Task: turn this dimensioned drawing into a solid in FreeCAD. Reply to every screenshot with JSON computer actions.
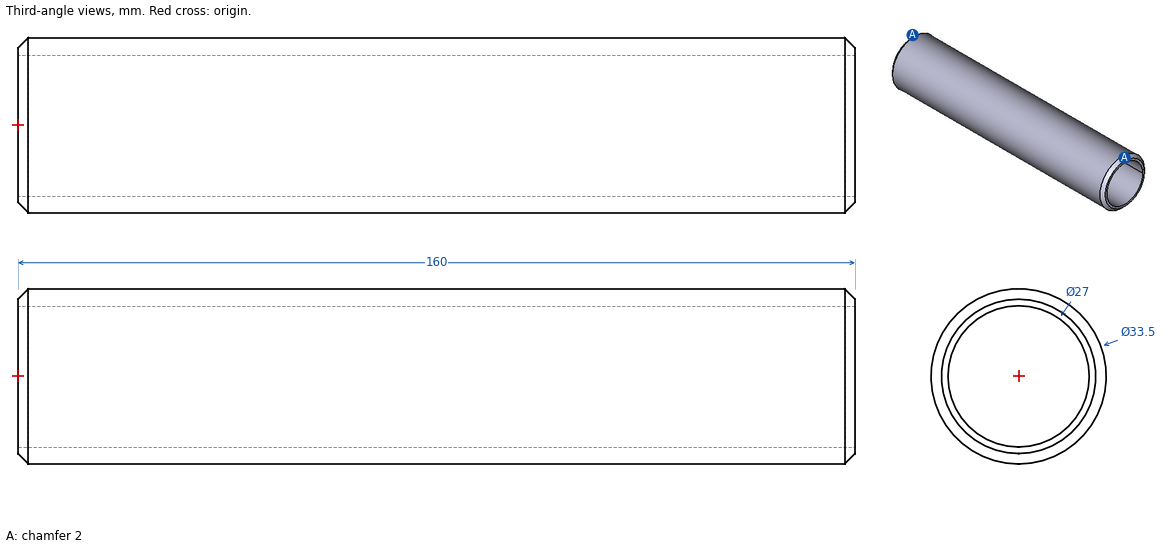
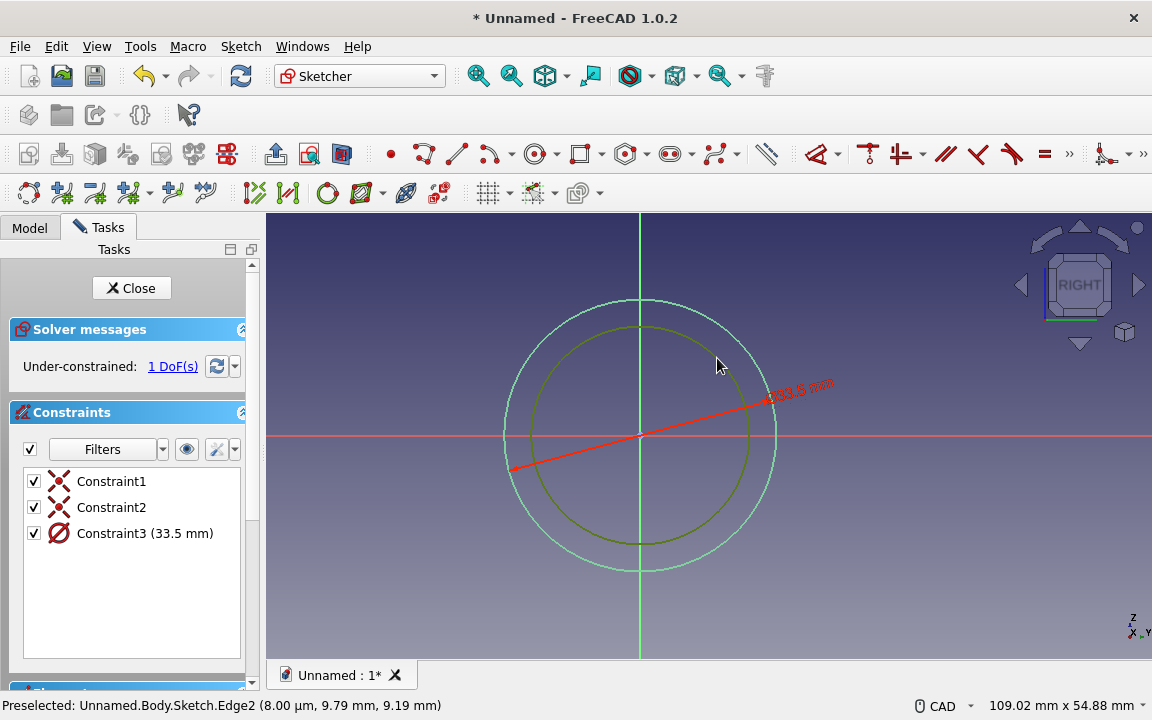
{"action": "key", "text": "k o"}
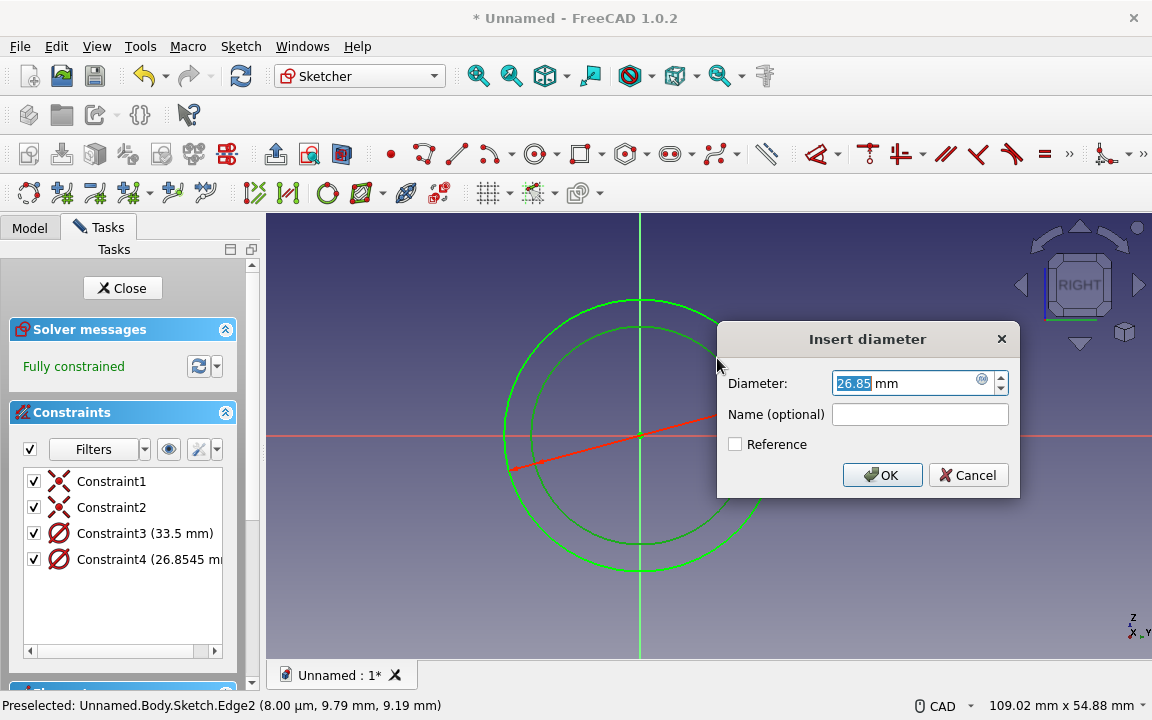
{"action": "type", "text": "27"}
{"action": "key", "text": "Return"}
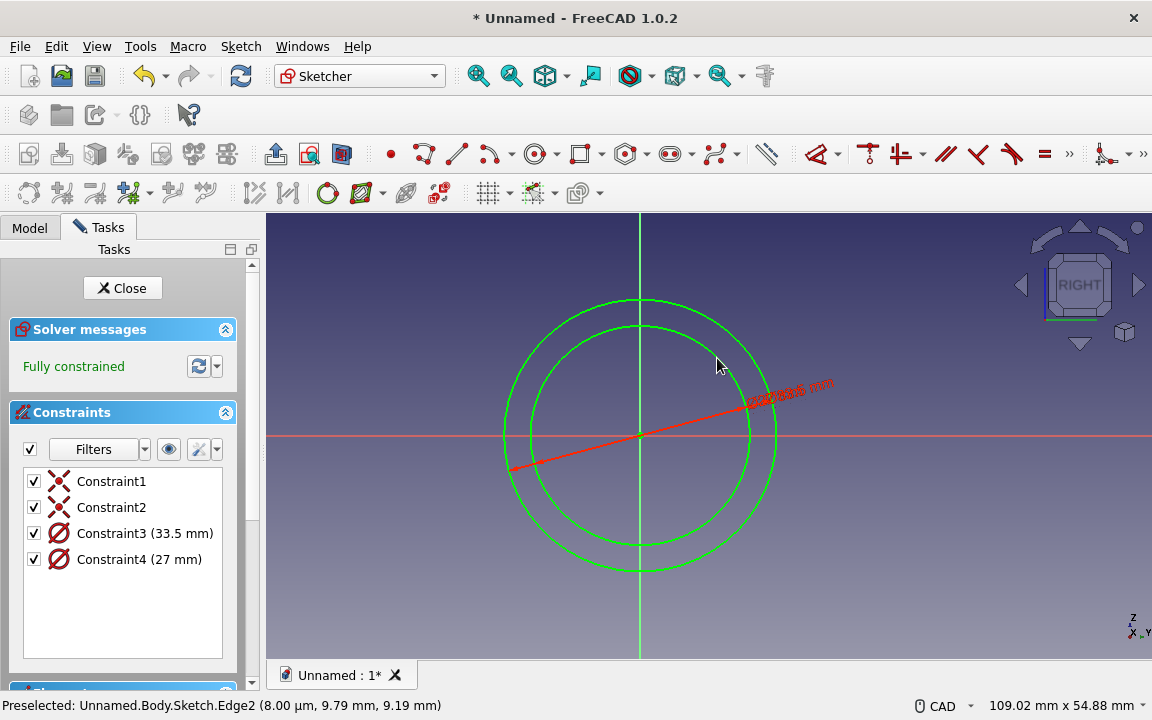
{"action": "left_click", "coordinate": [123, 288]}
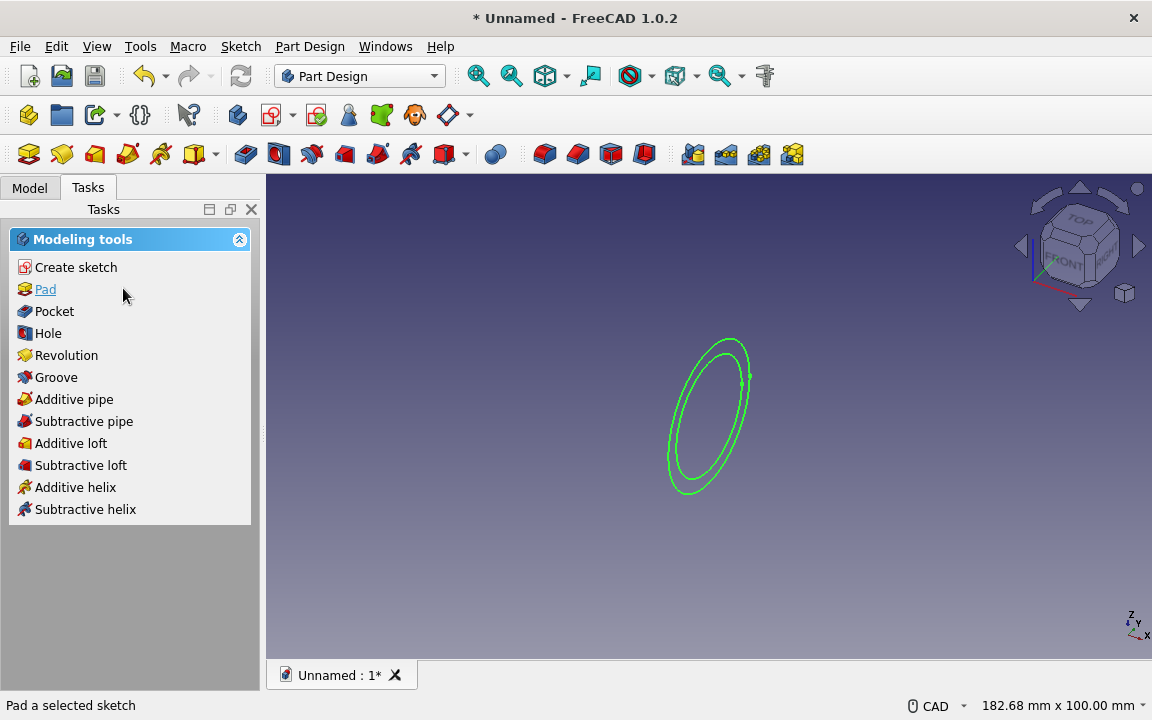
{"action": "left_click", "coordinate": [29, 154]}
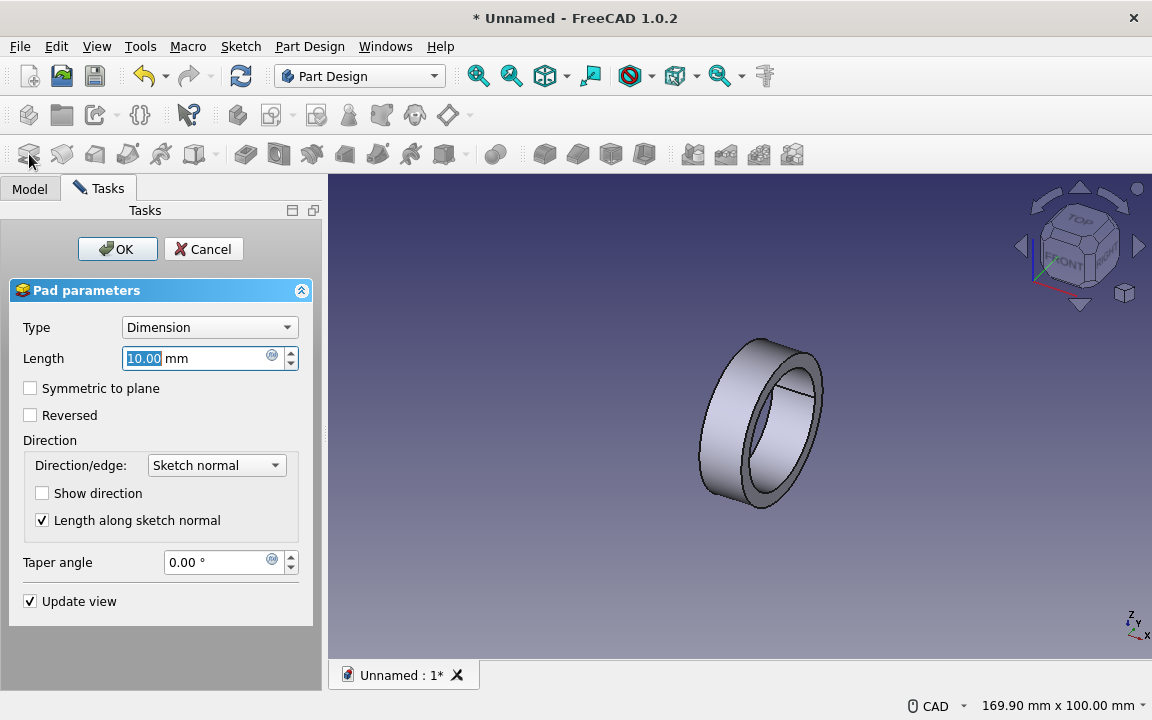
{"action": "type", "text": "160"}
{"action": "key", "text": "Tab"}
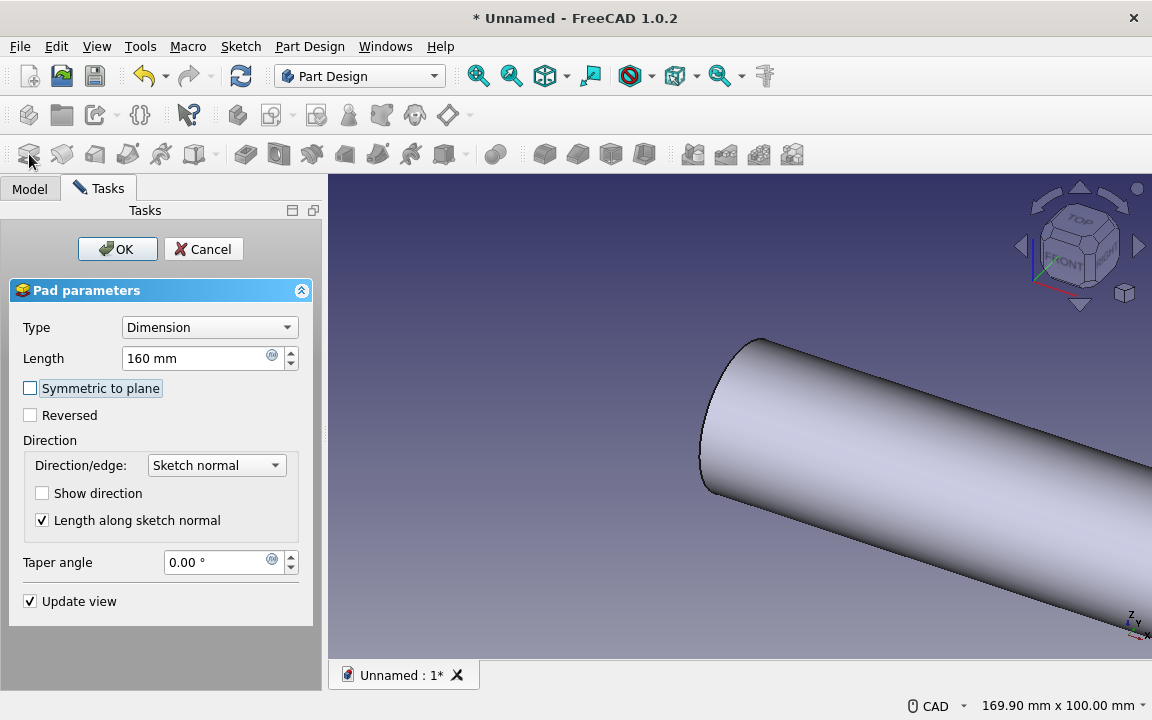
{"action": "left_click", "coordinate": [118, 249]}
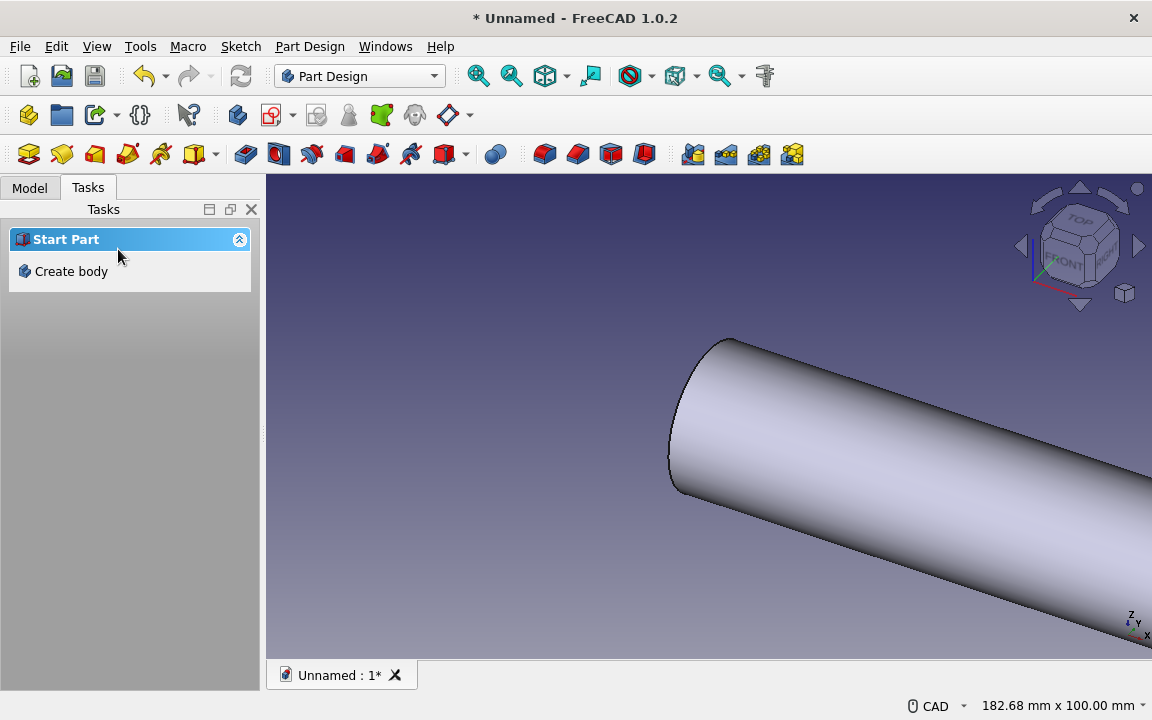
{"action": "key", "text": "v f"}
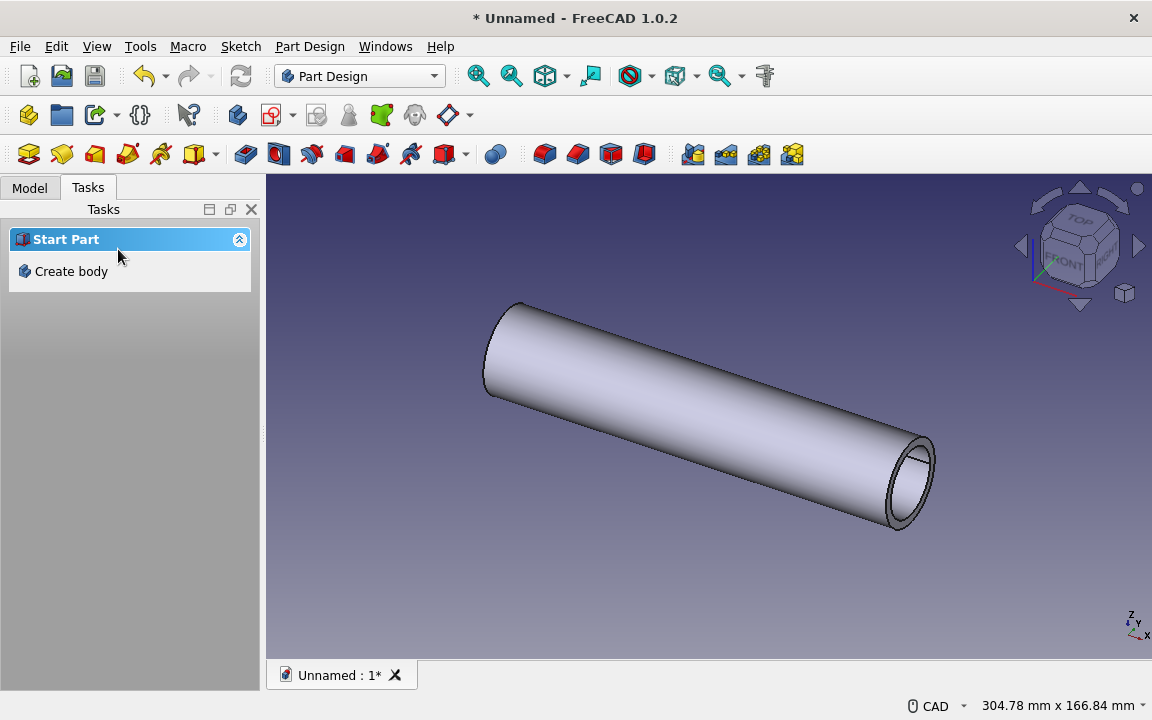
{"action": "left_click", "coordinate": [886, 506]}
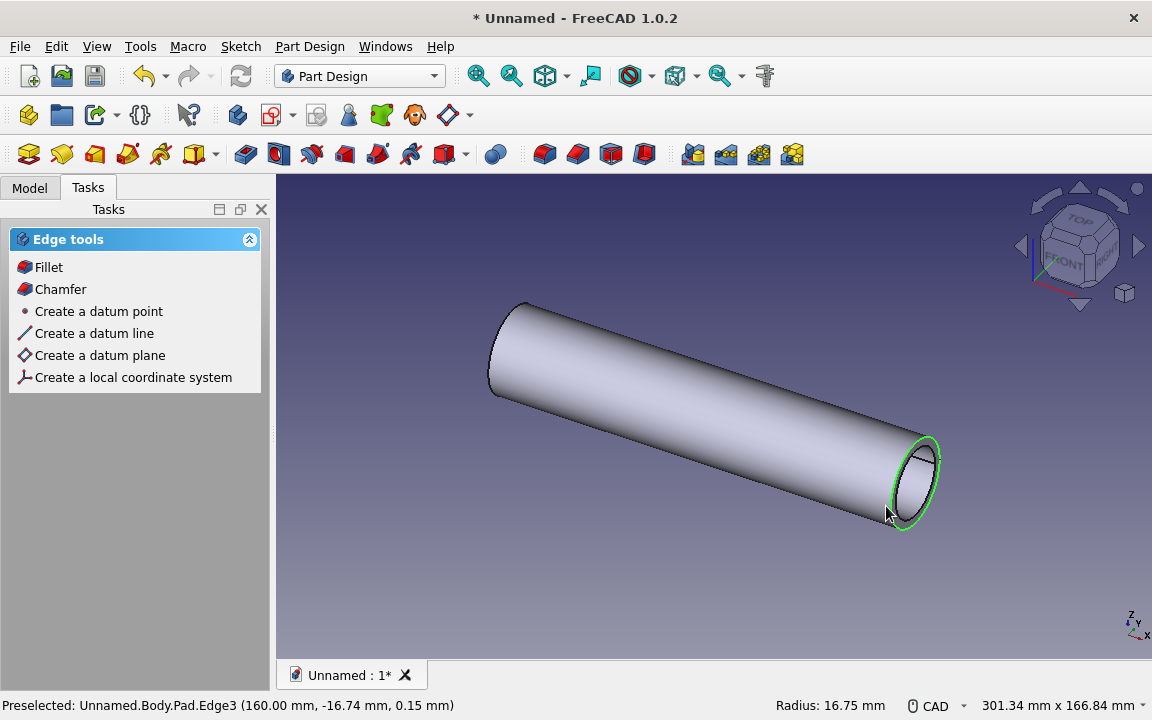
{"action": "key", "text": "0"}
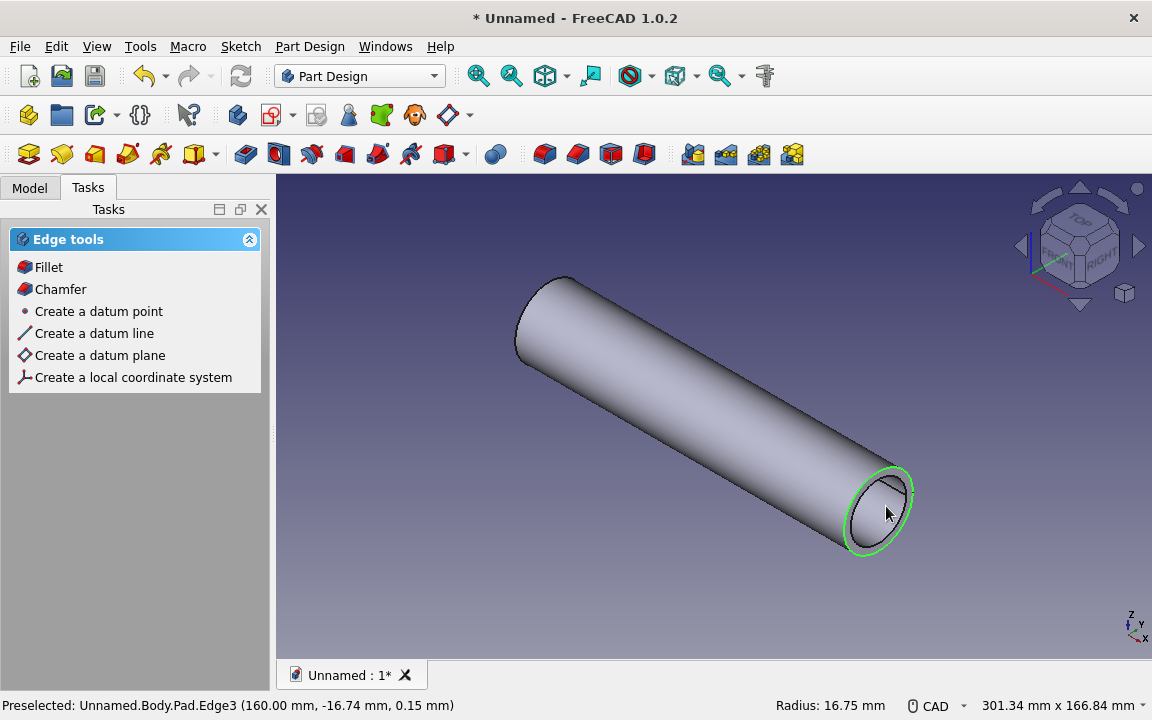
{"action": "key", "text": "2"}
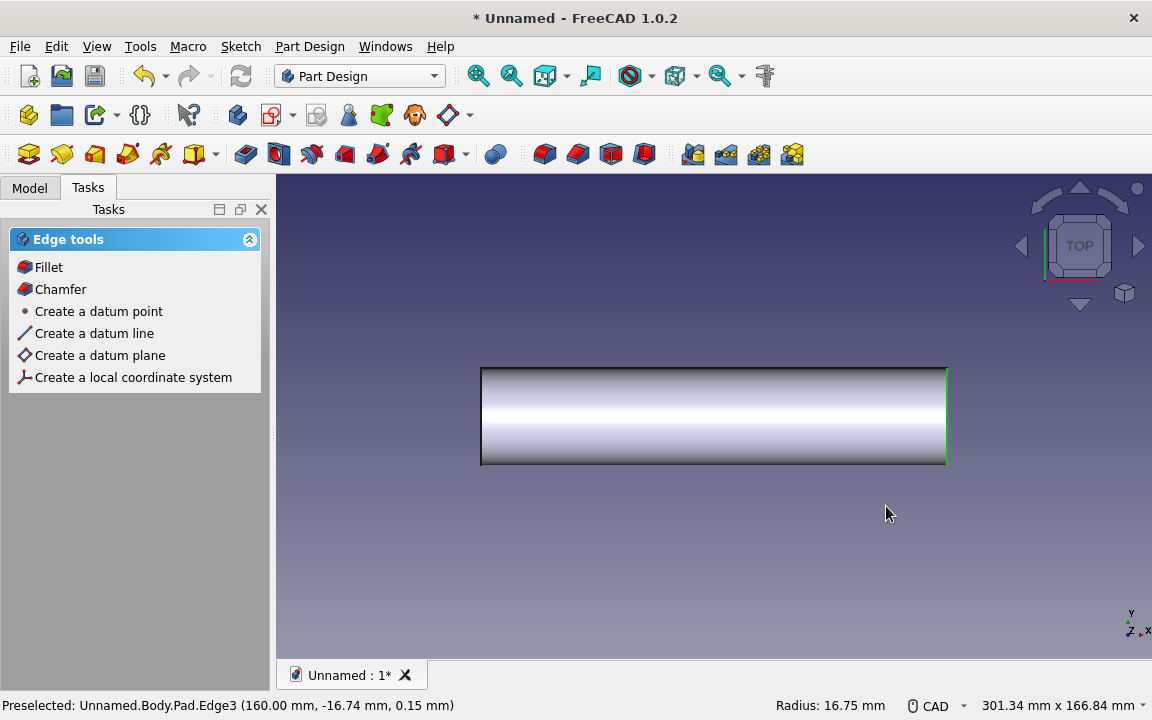
{"action": "left_click", "coordinate": [481, 455], "text": "ctrl"}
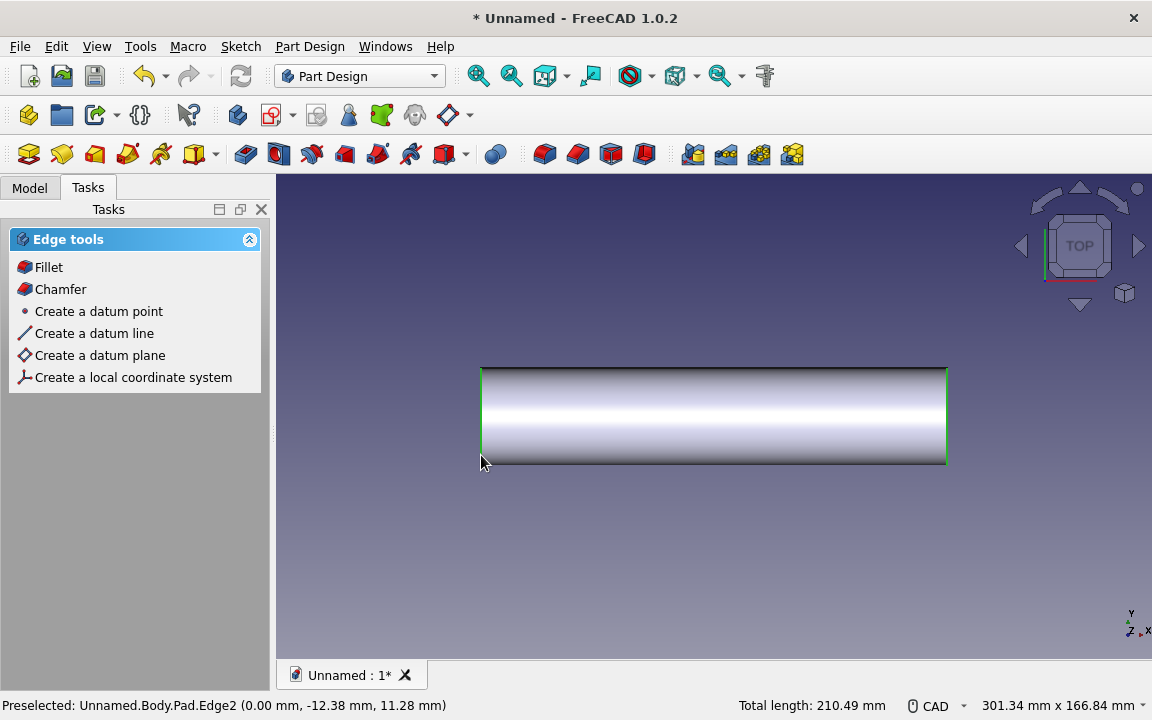
{"action": "left_click", "coordinate": [578, 154]}